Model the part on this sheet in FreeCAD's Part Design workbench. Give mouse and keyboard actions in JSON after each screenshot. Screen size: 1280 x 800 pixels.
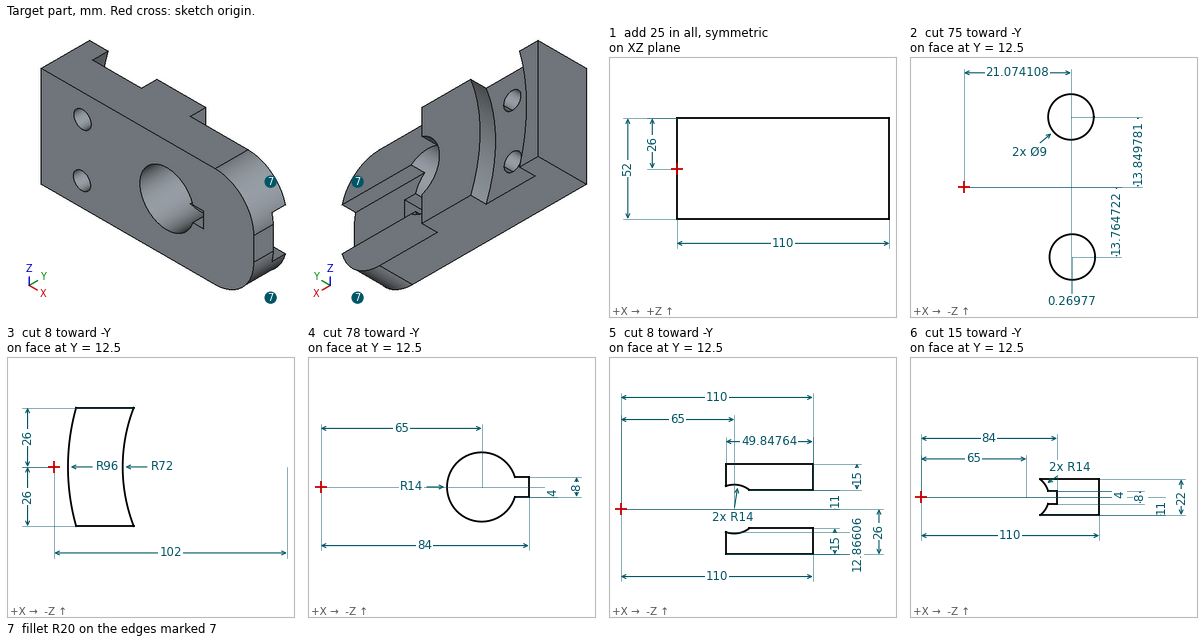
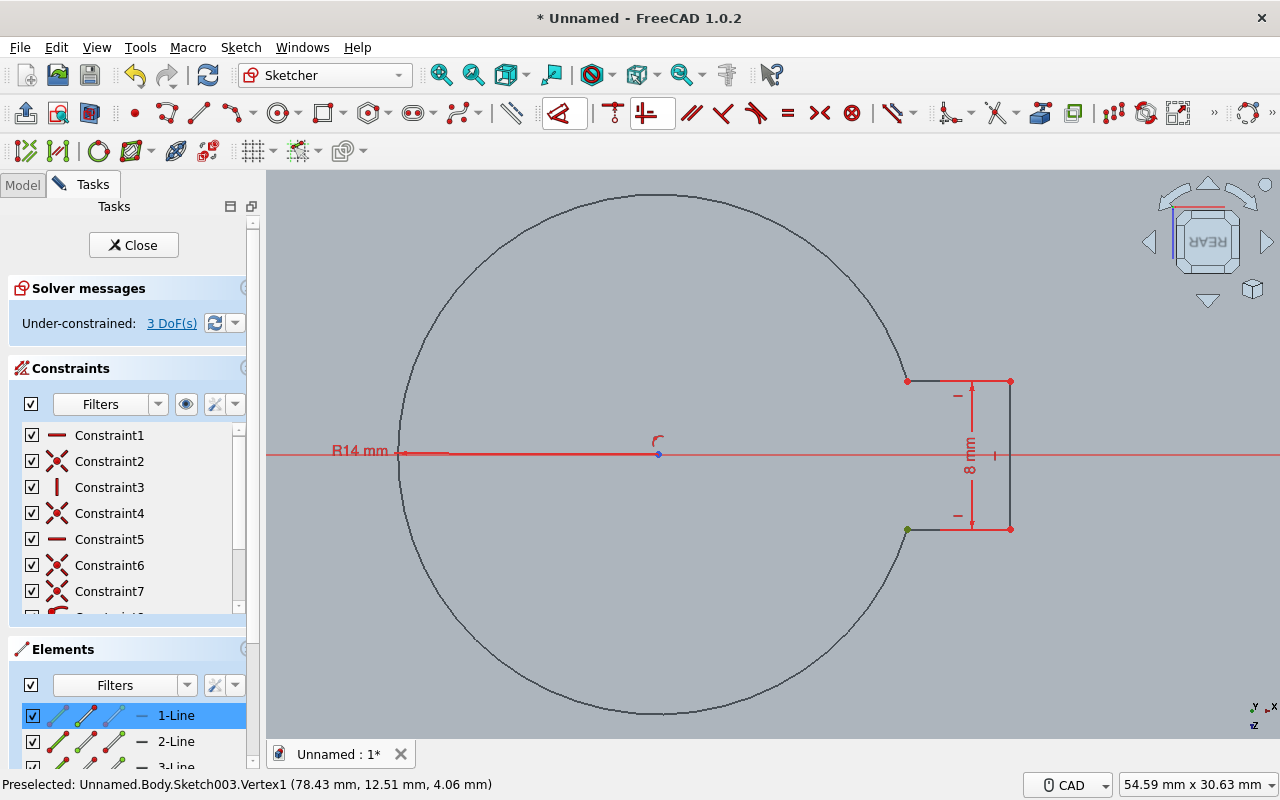
{"action": "left_click", "coordinate": [582, 114]}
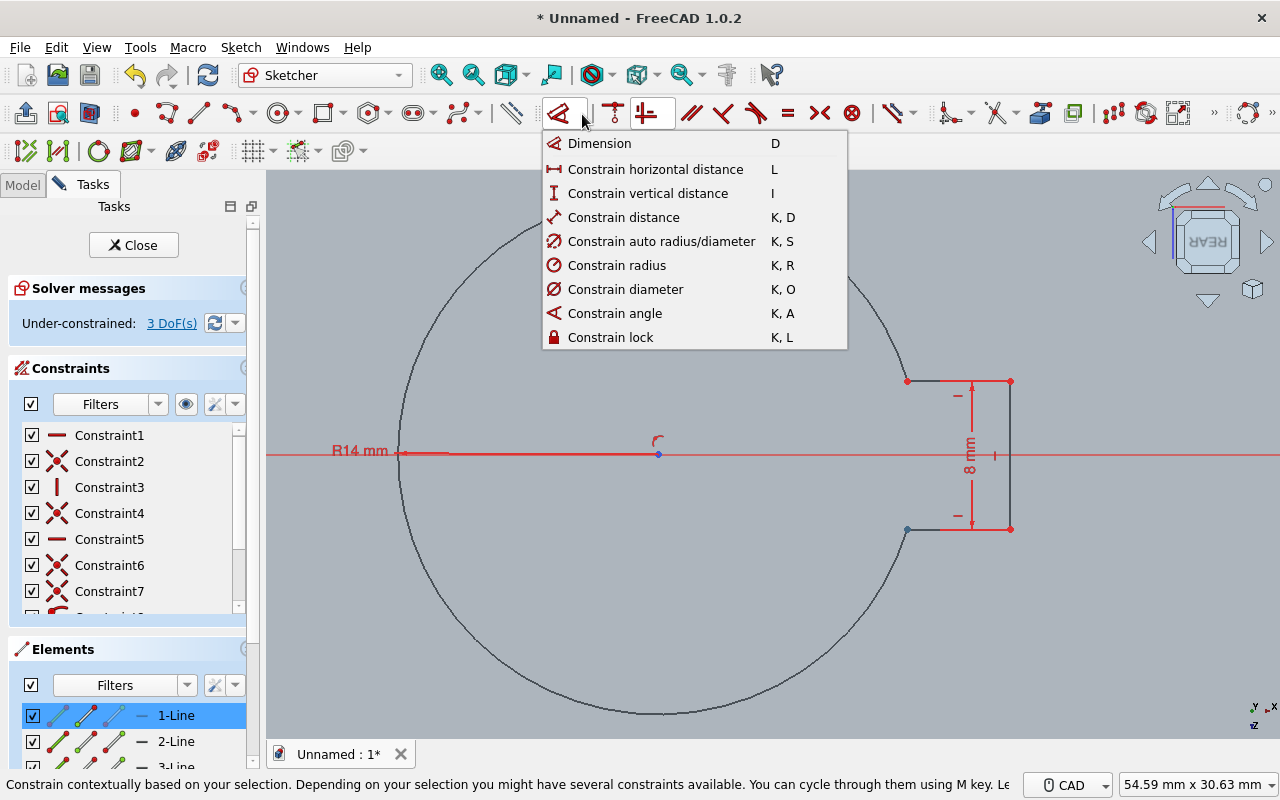
{"action": "left_click", "coordinate": [695, 193]}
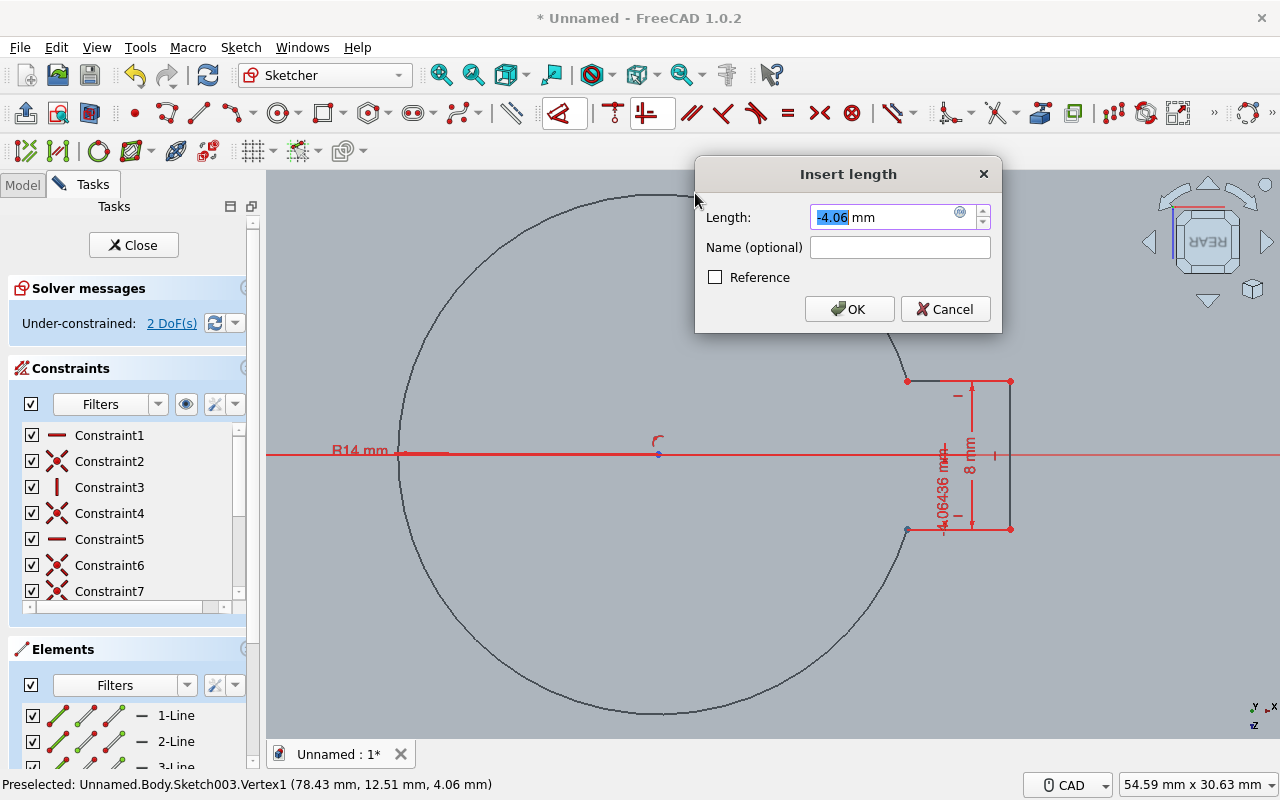
{"action": "type", "text": "-4"}
{"action": "key", "text": "Return"}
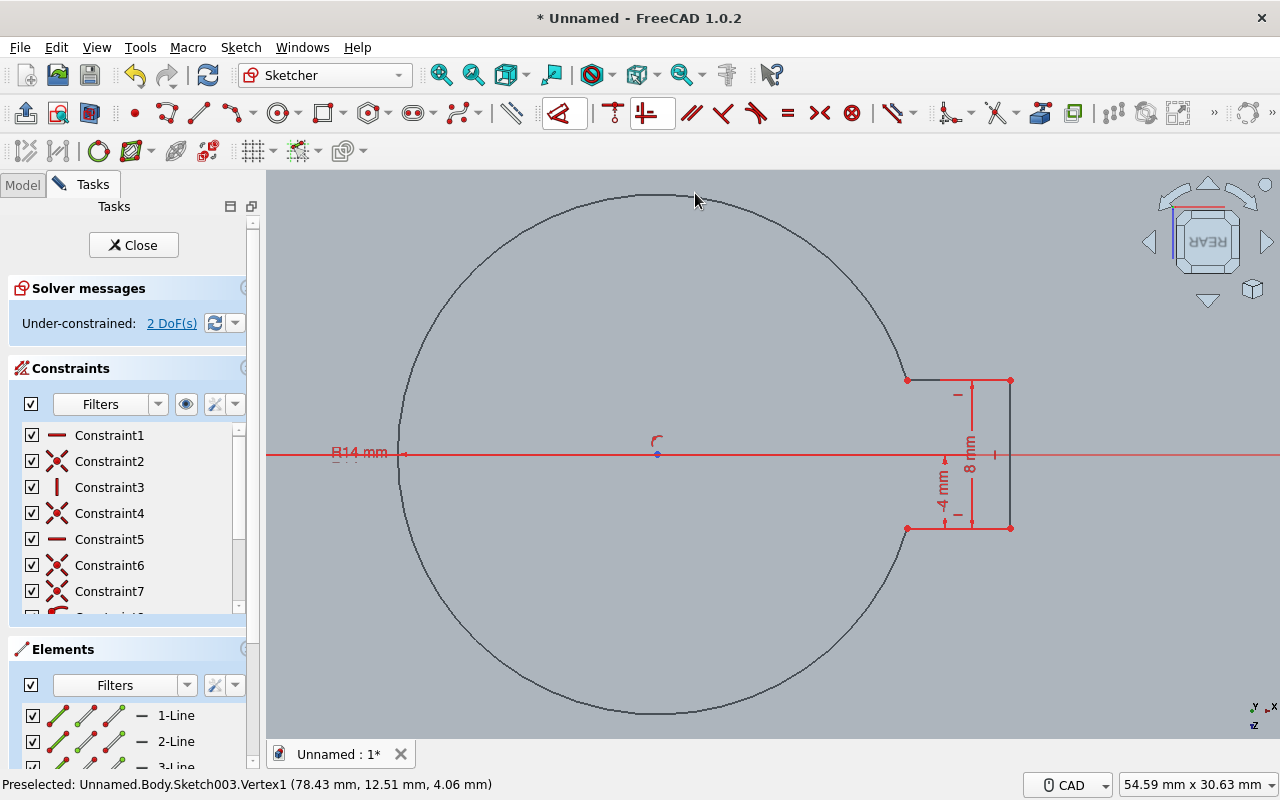
{"action": "left_click", "coordinate": [1010, 529]}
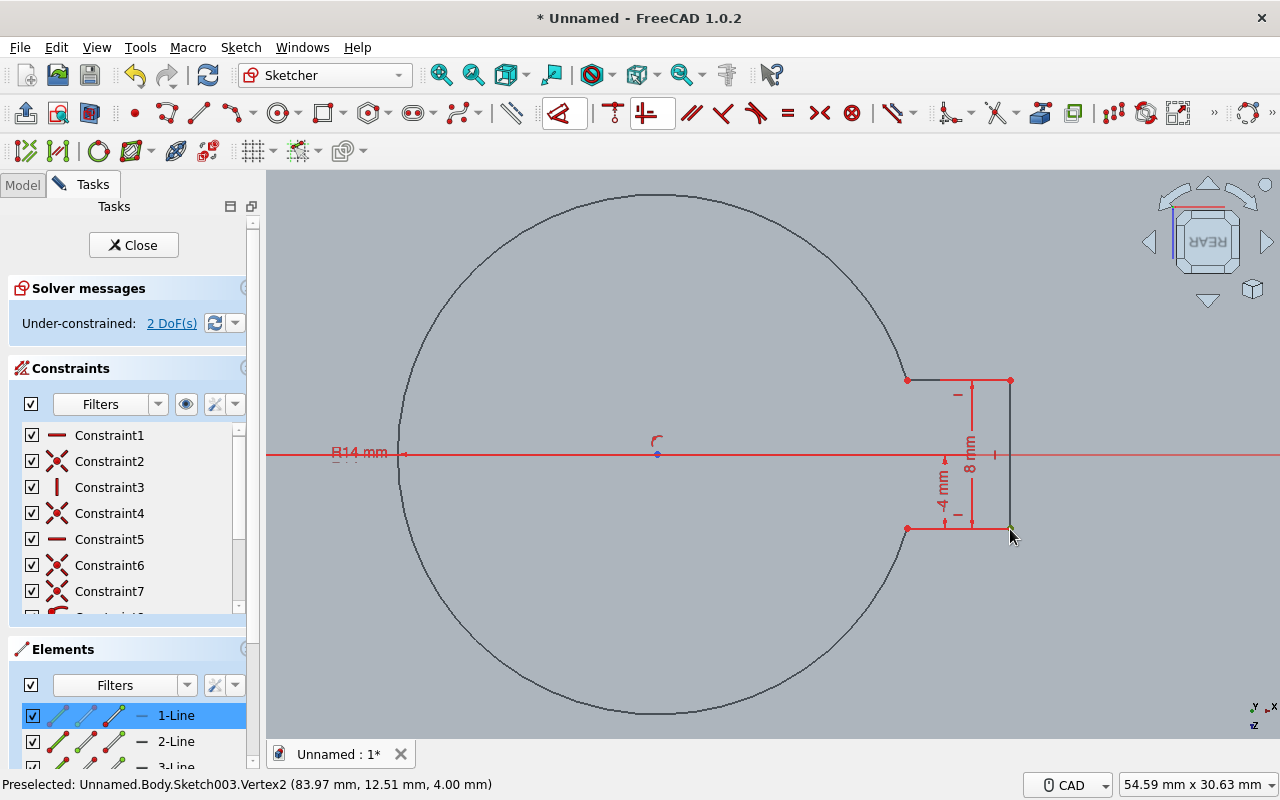
{"action": "key", "text": "l"}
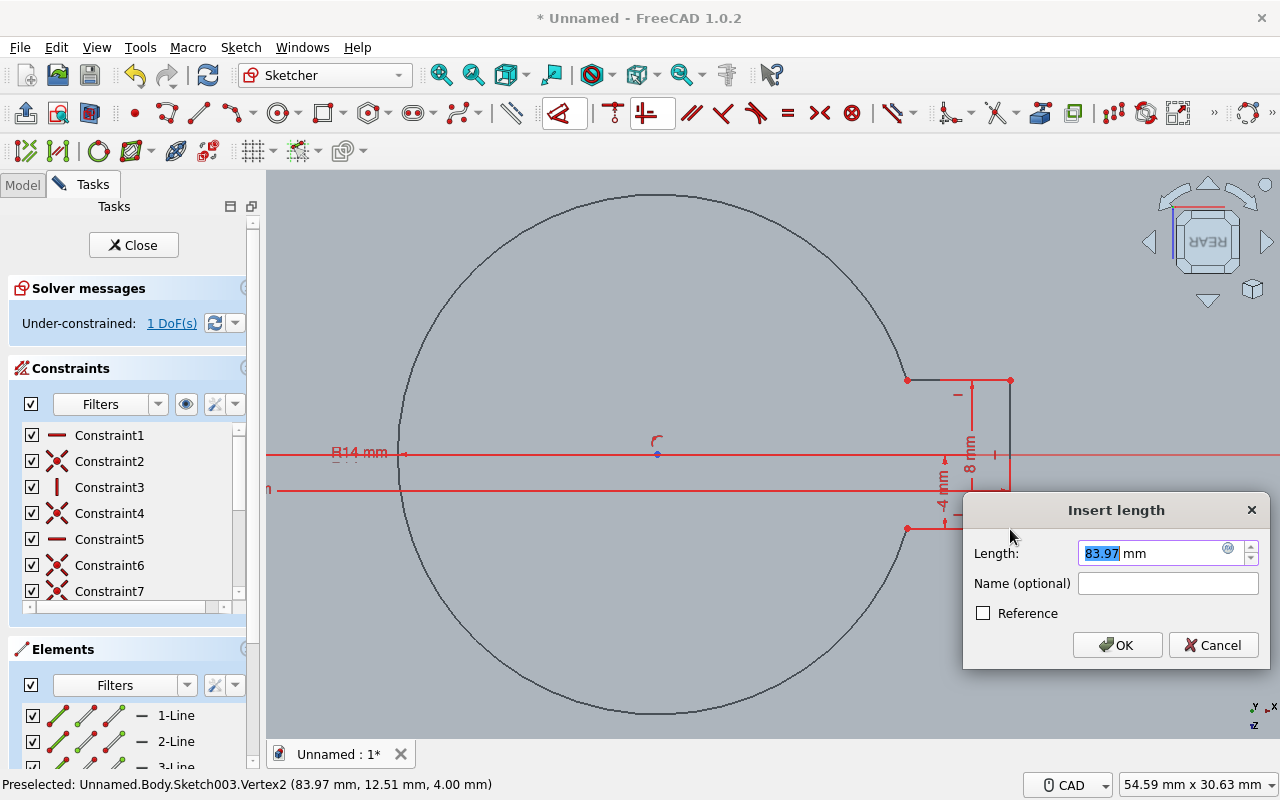
{"action": "type", "text": "84"}
{"action": "key", "text": "Return"}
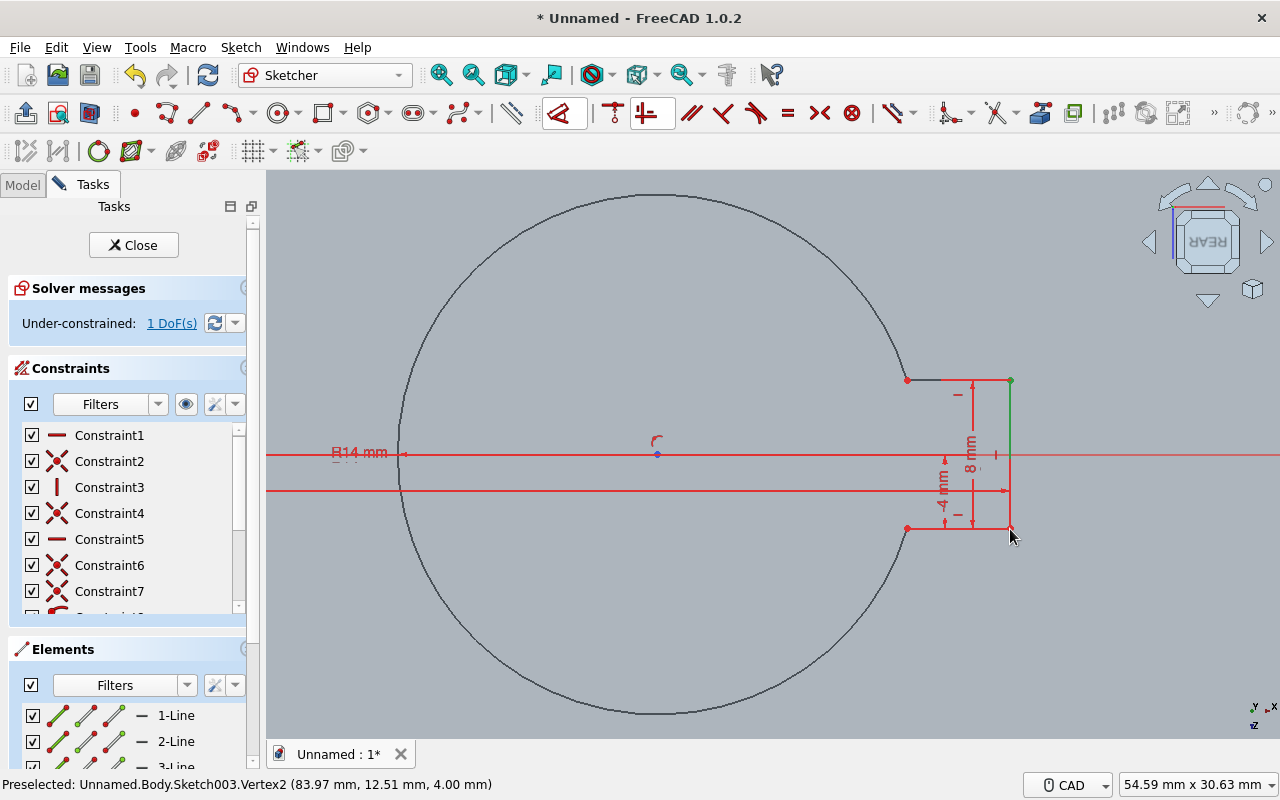
{"action": "left_click", "coordinate": [658, 454]}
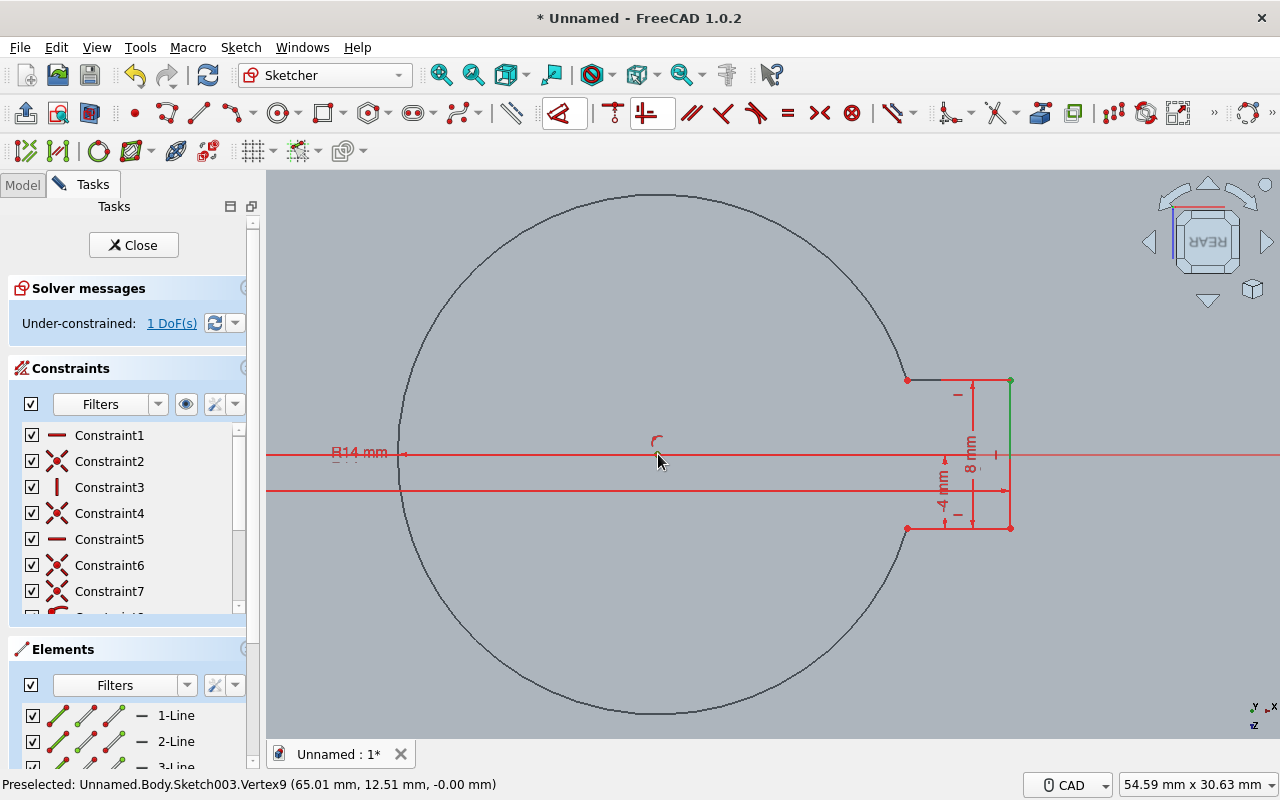
{"action": "key", "text": "l"}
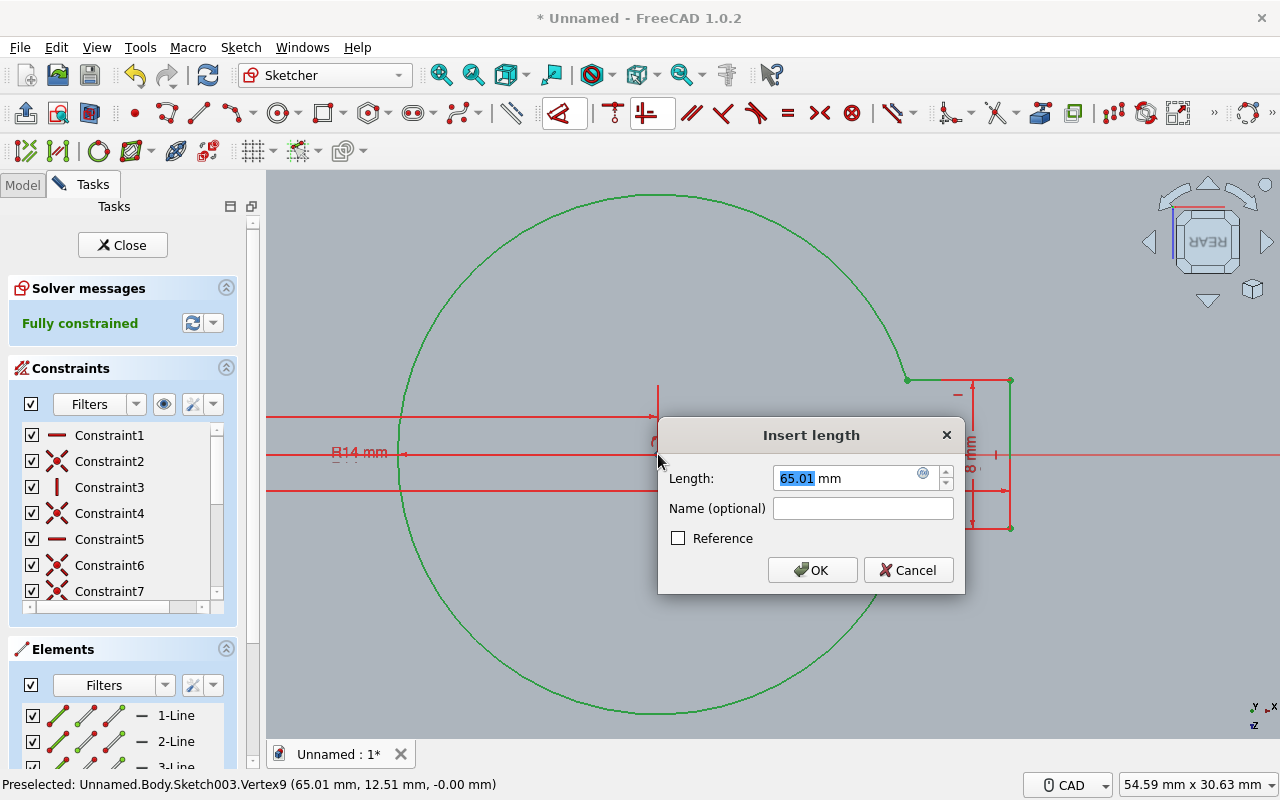
{"action": "type", "text": "65"}
{"action": "key", "text": "Return"}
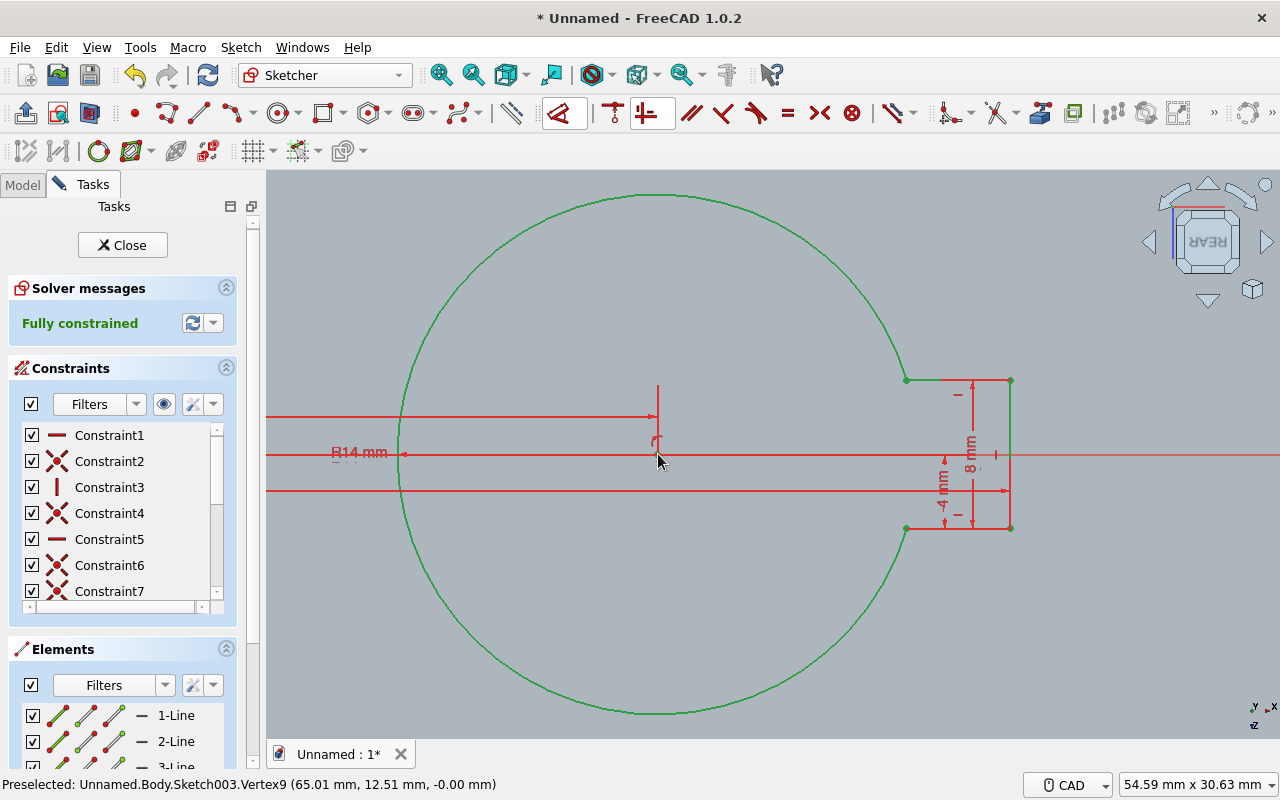
{"action": "left_click", "coordinate": [123, 245]}